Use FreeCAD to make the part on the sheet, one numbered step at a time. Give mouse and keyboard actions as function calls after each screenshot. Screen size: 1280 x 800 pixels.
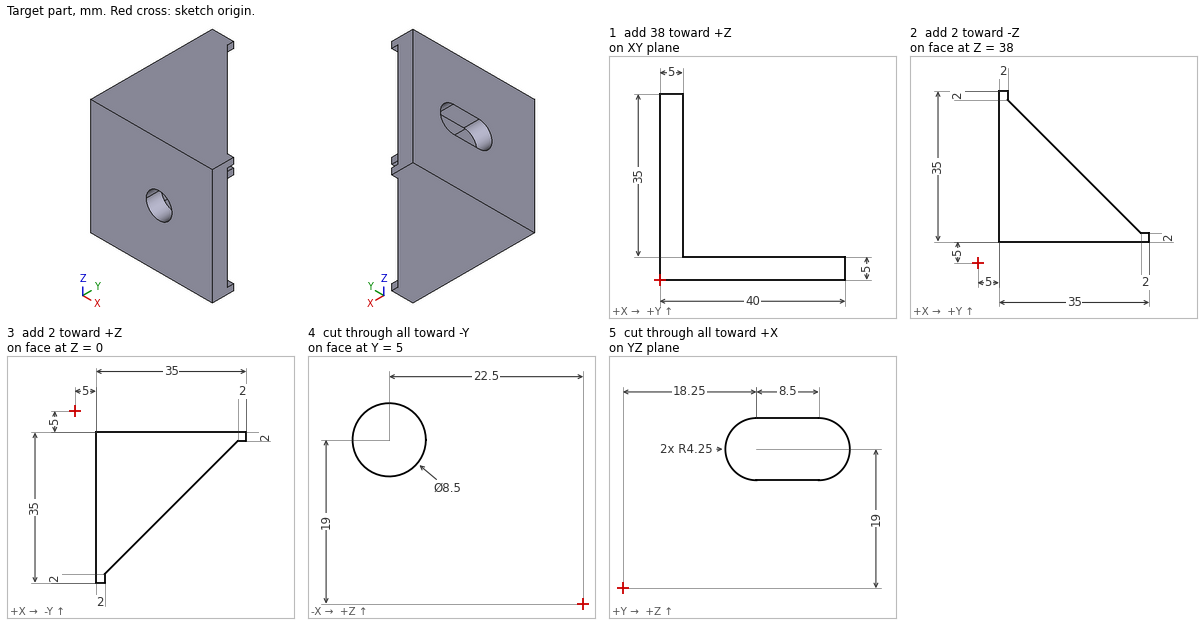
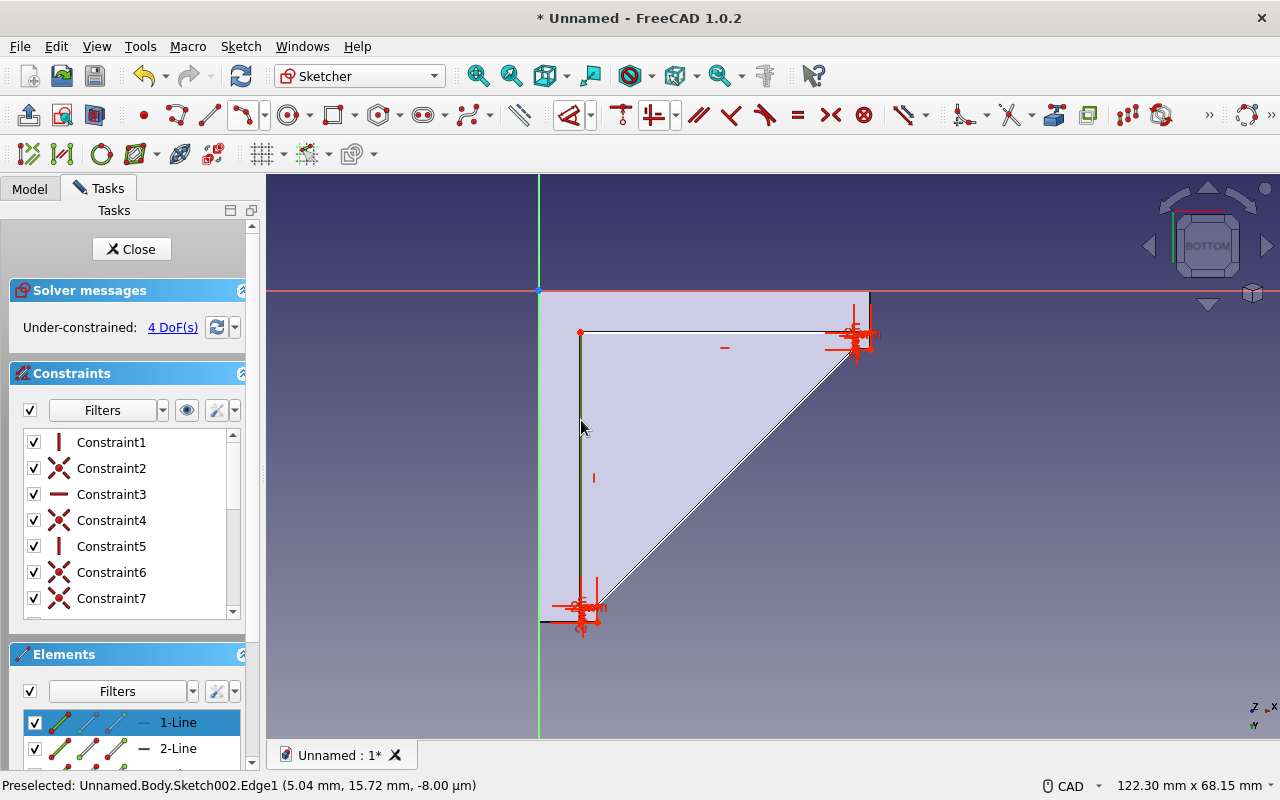
key(i)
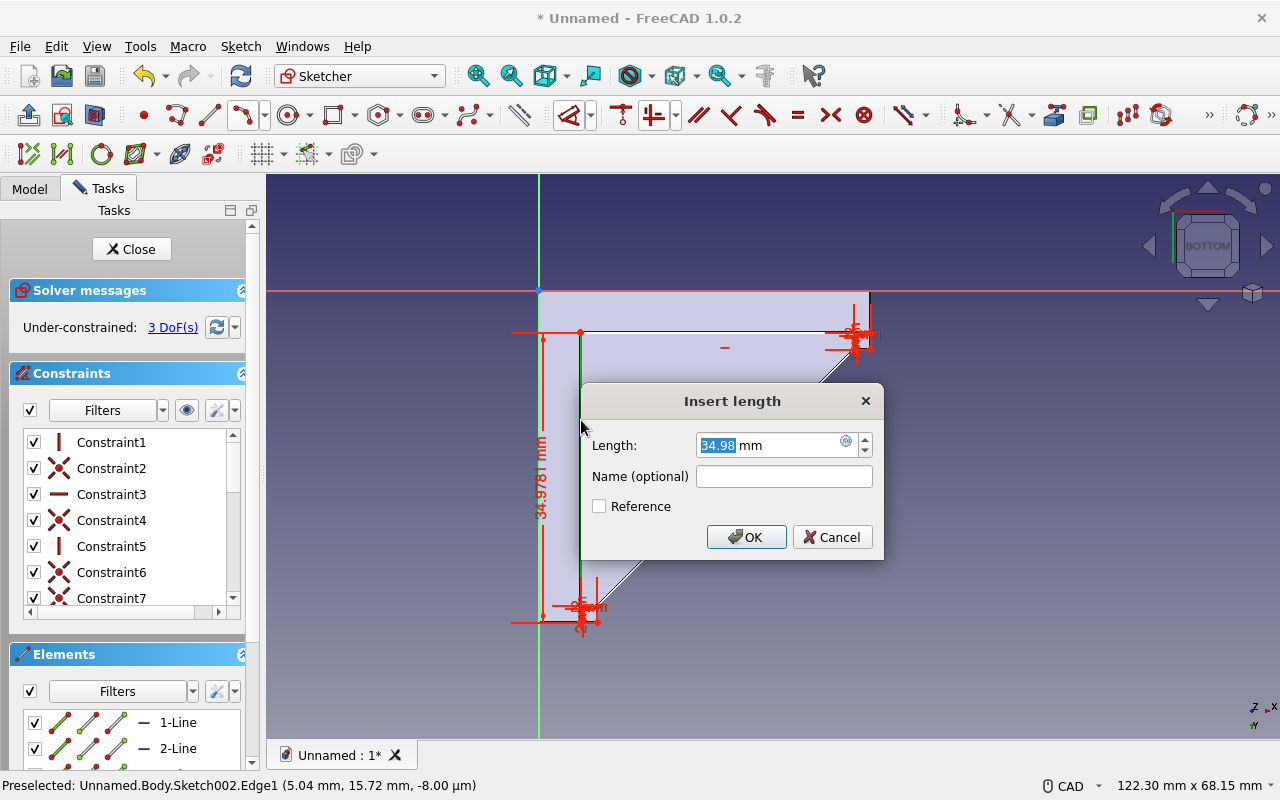
text(35)
key(Return)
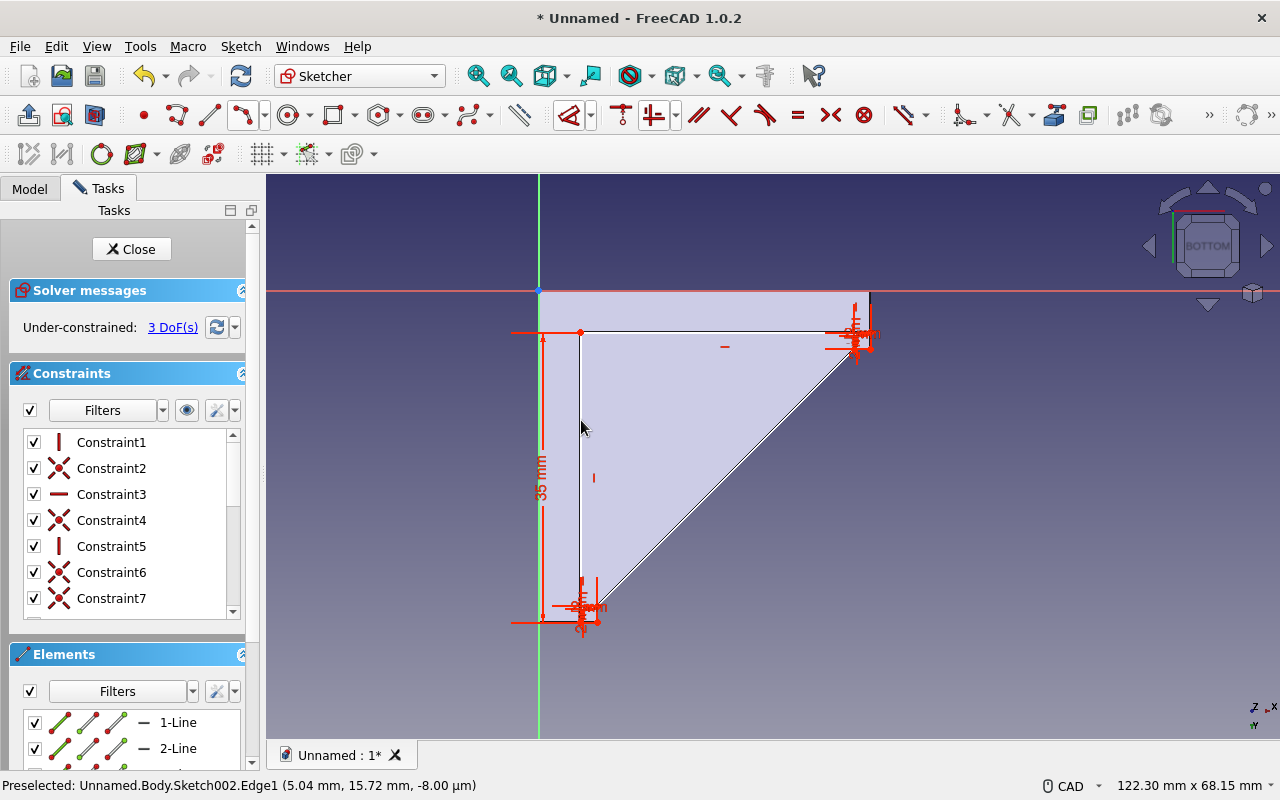
click(784, 333)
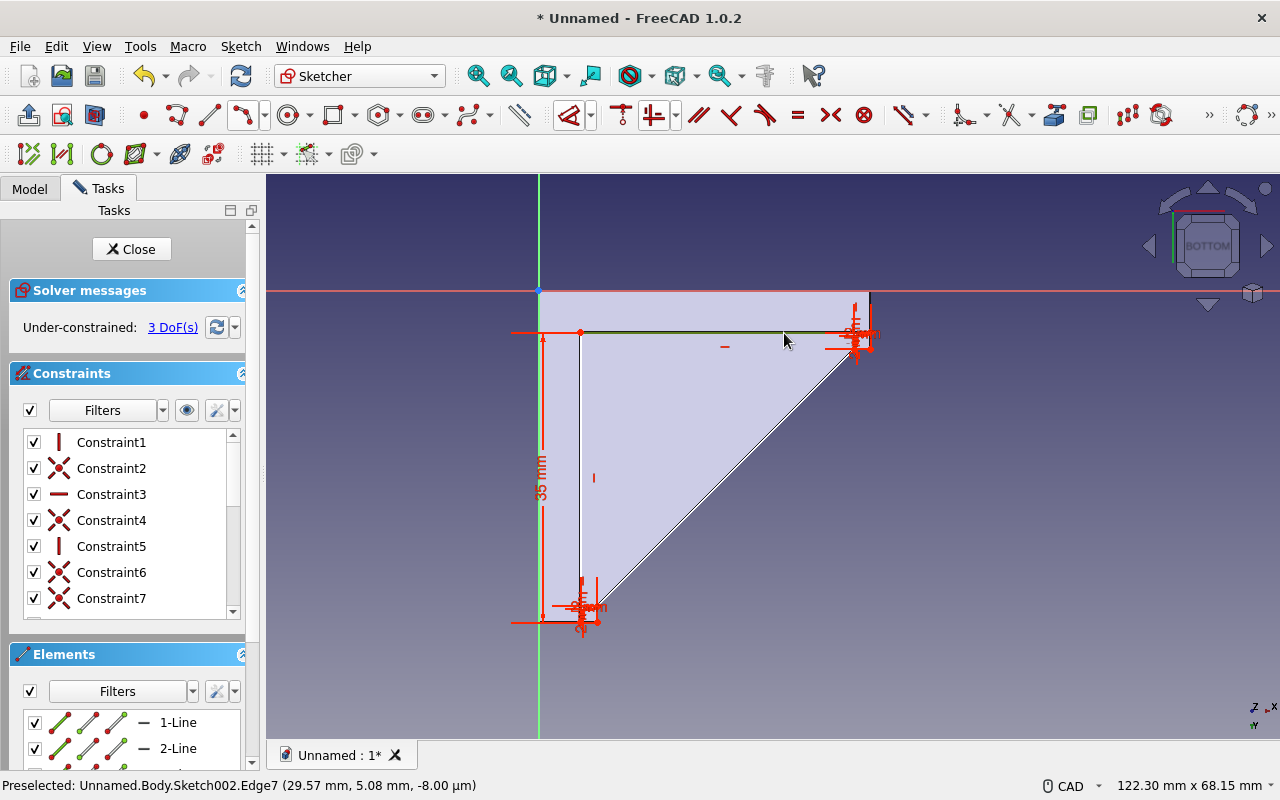
key(l)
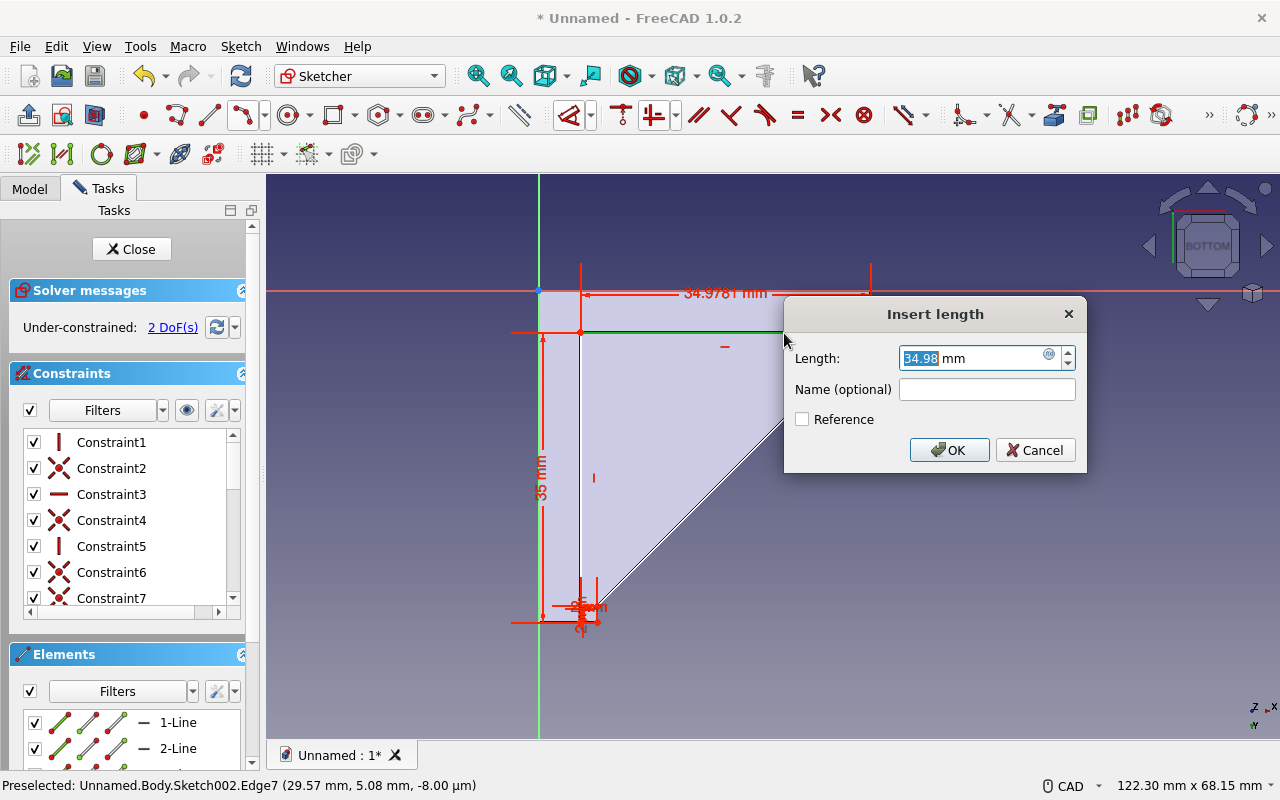
text(35)
key(Return)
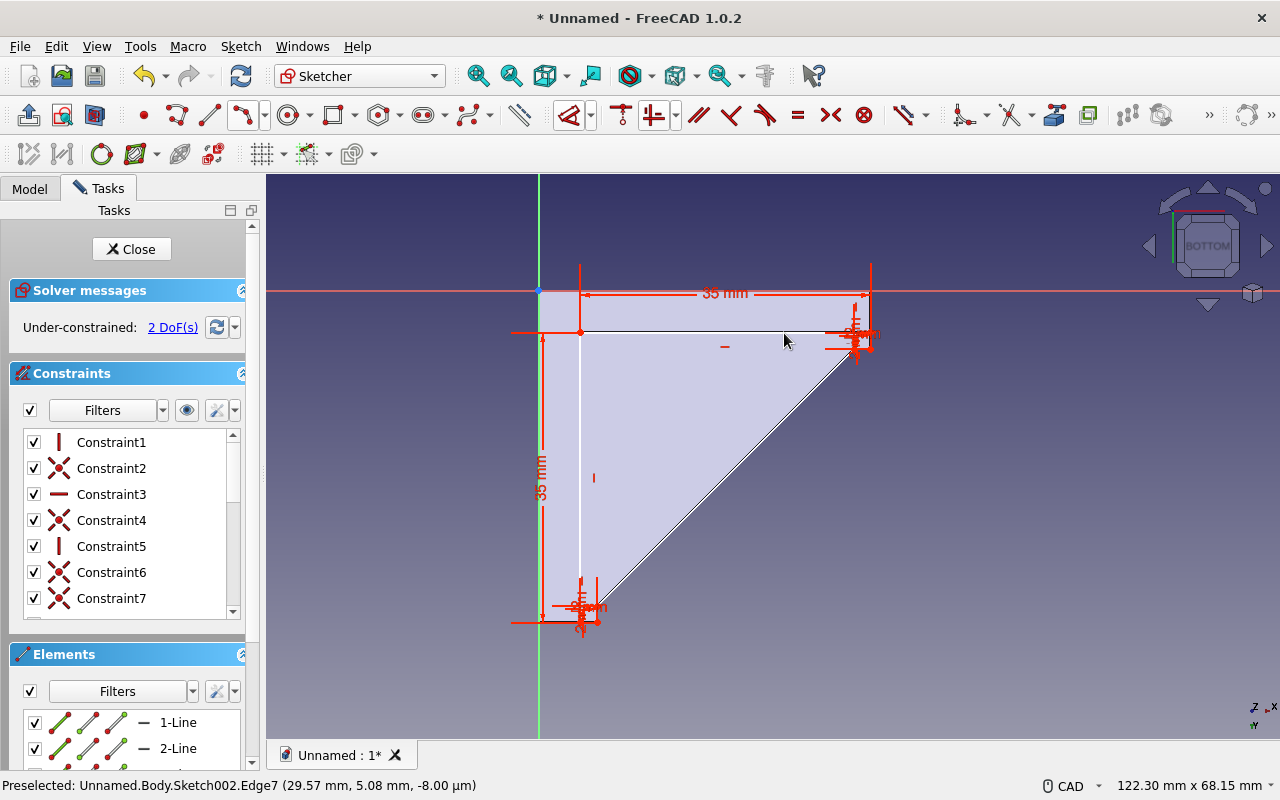
click(580, 333)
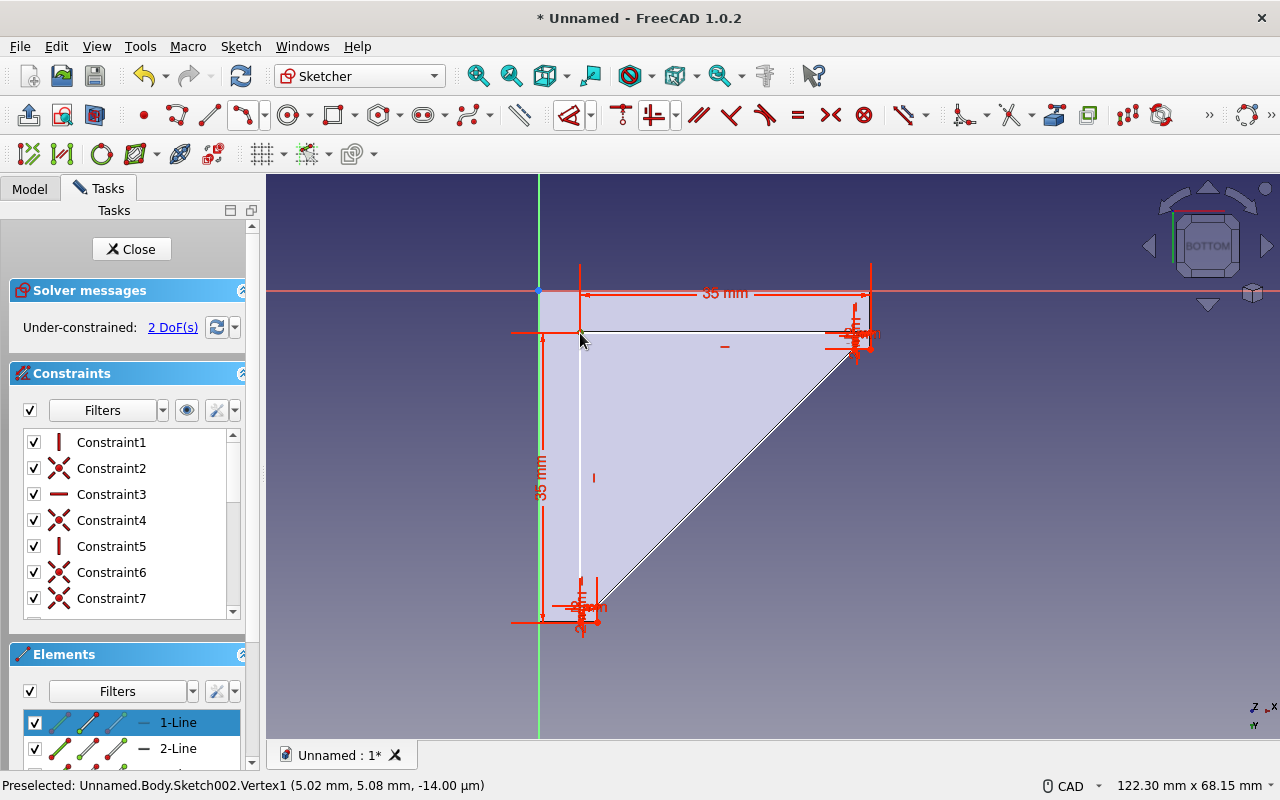
key(l)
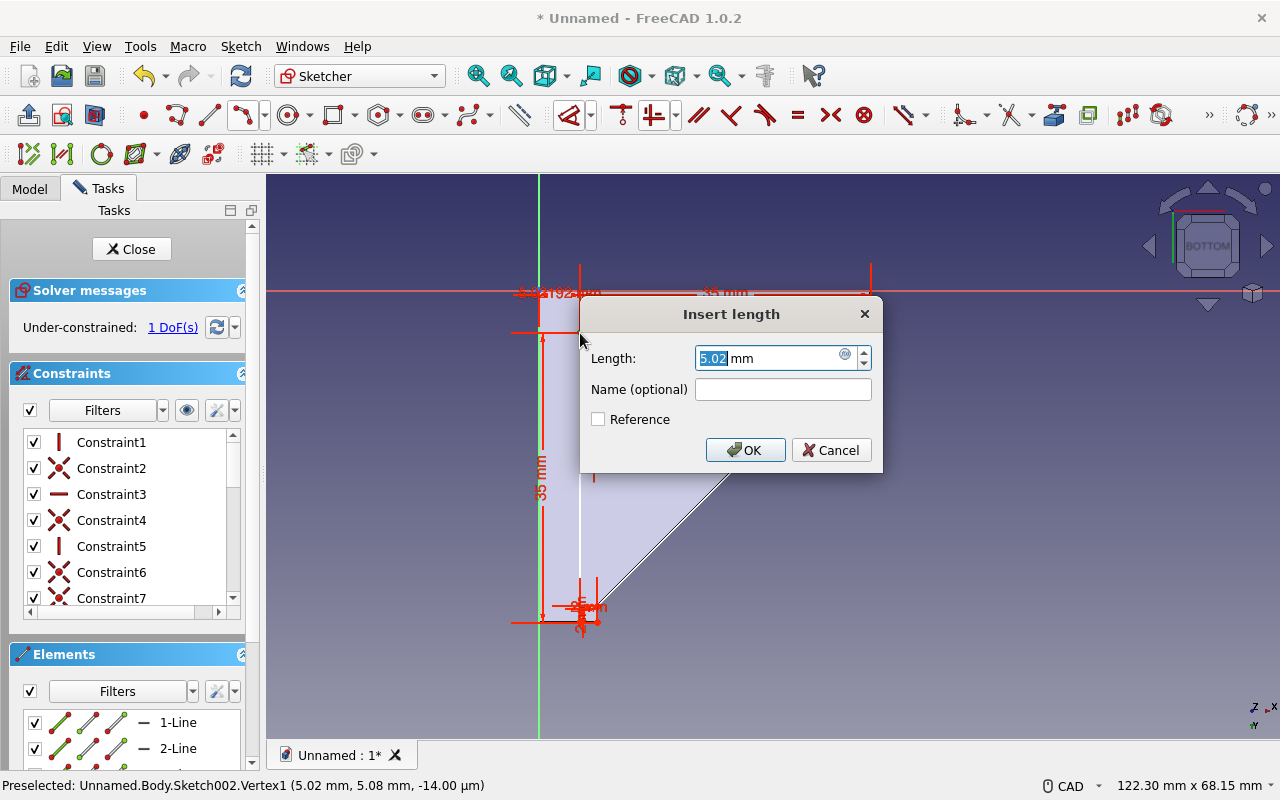
text(5)
key(Return)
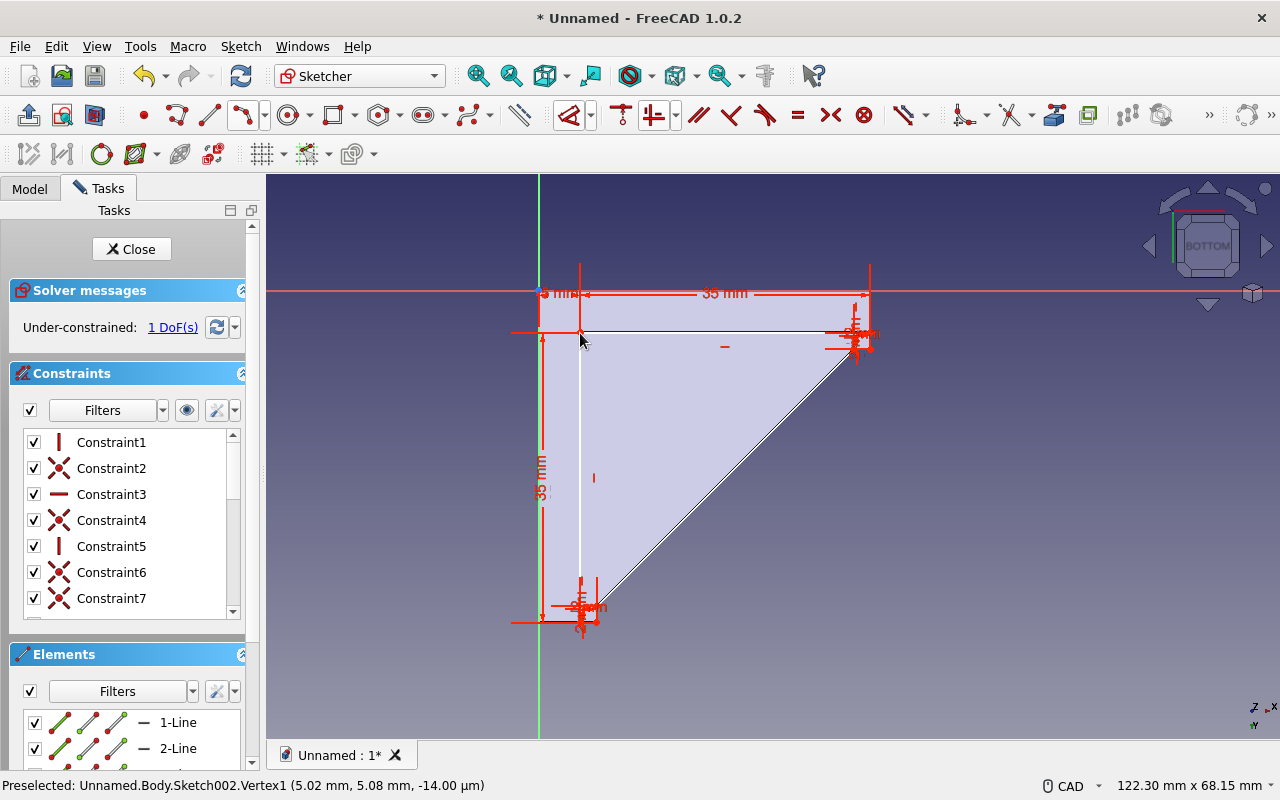
click(580, 333)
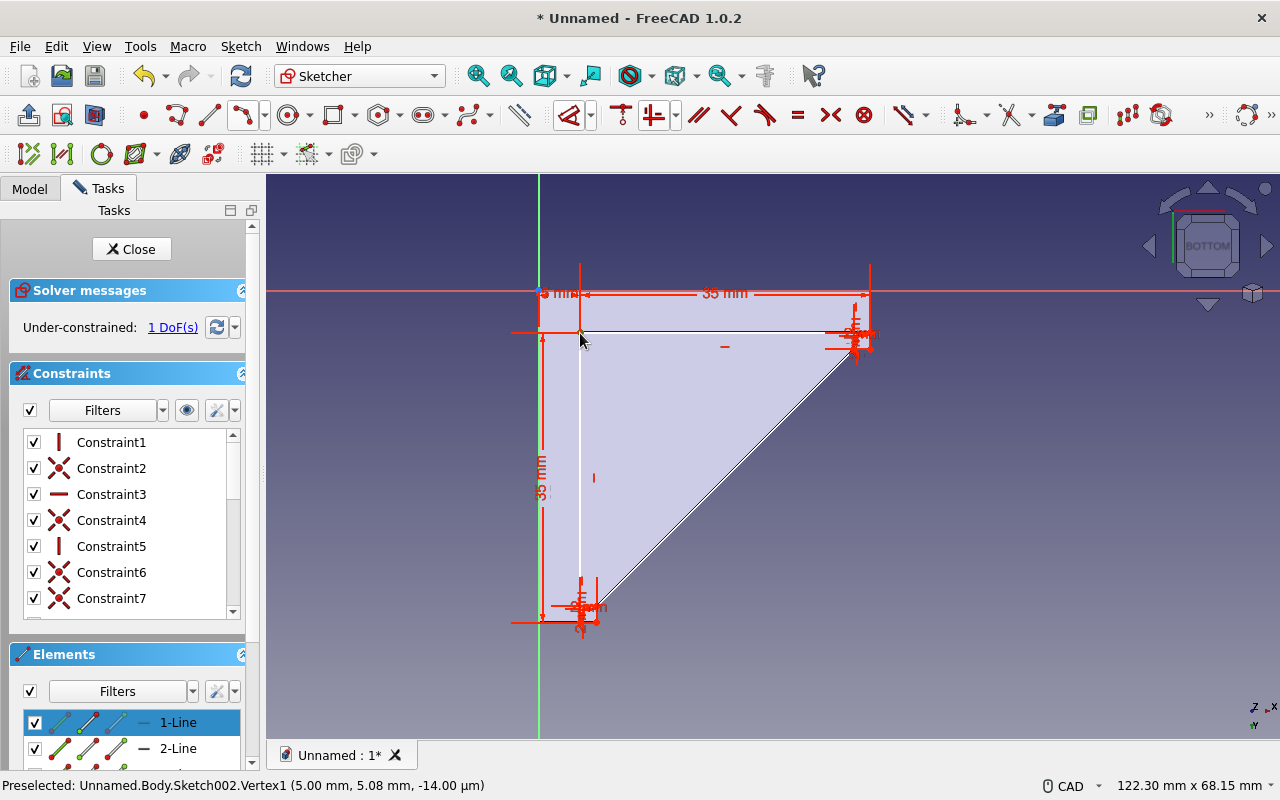
key(i)